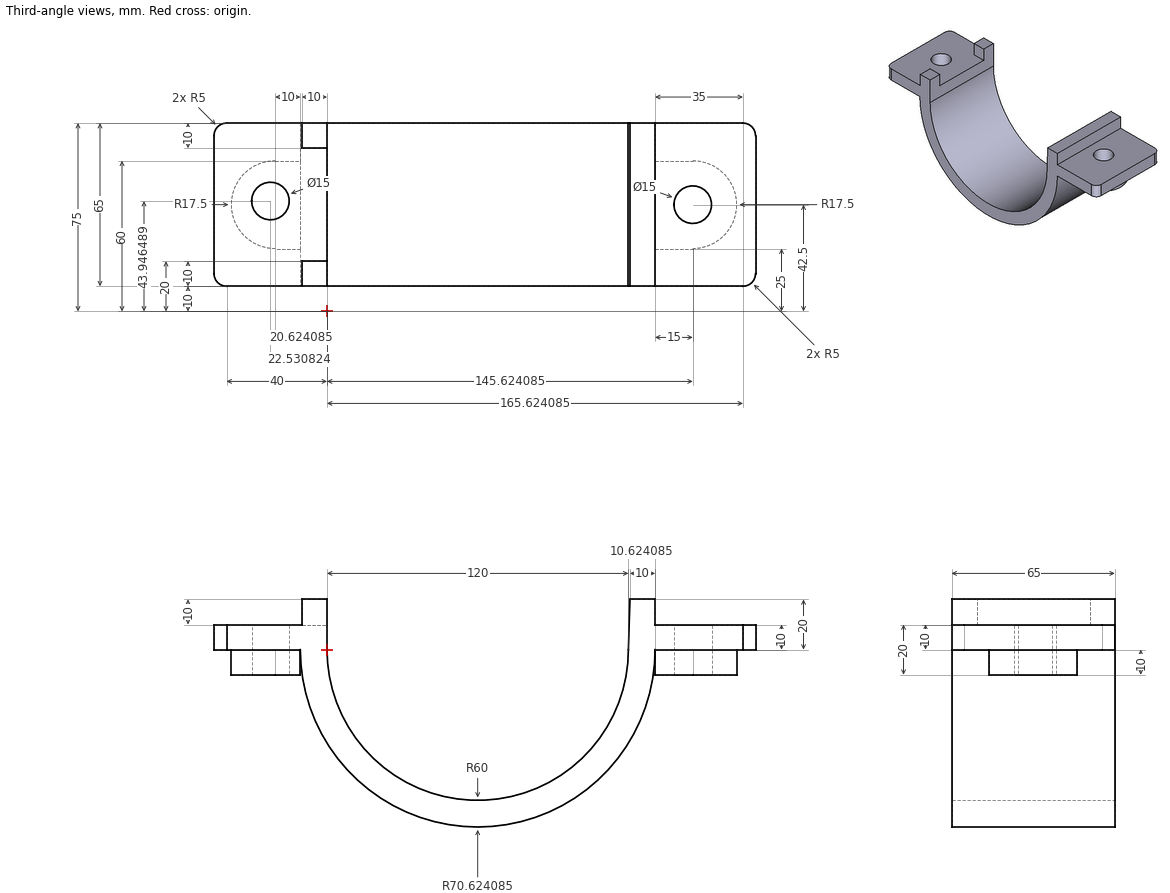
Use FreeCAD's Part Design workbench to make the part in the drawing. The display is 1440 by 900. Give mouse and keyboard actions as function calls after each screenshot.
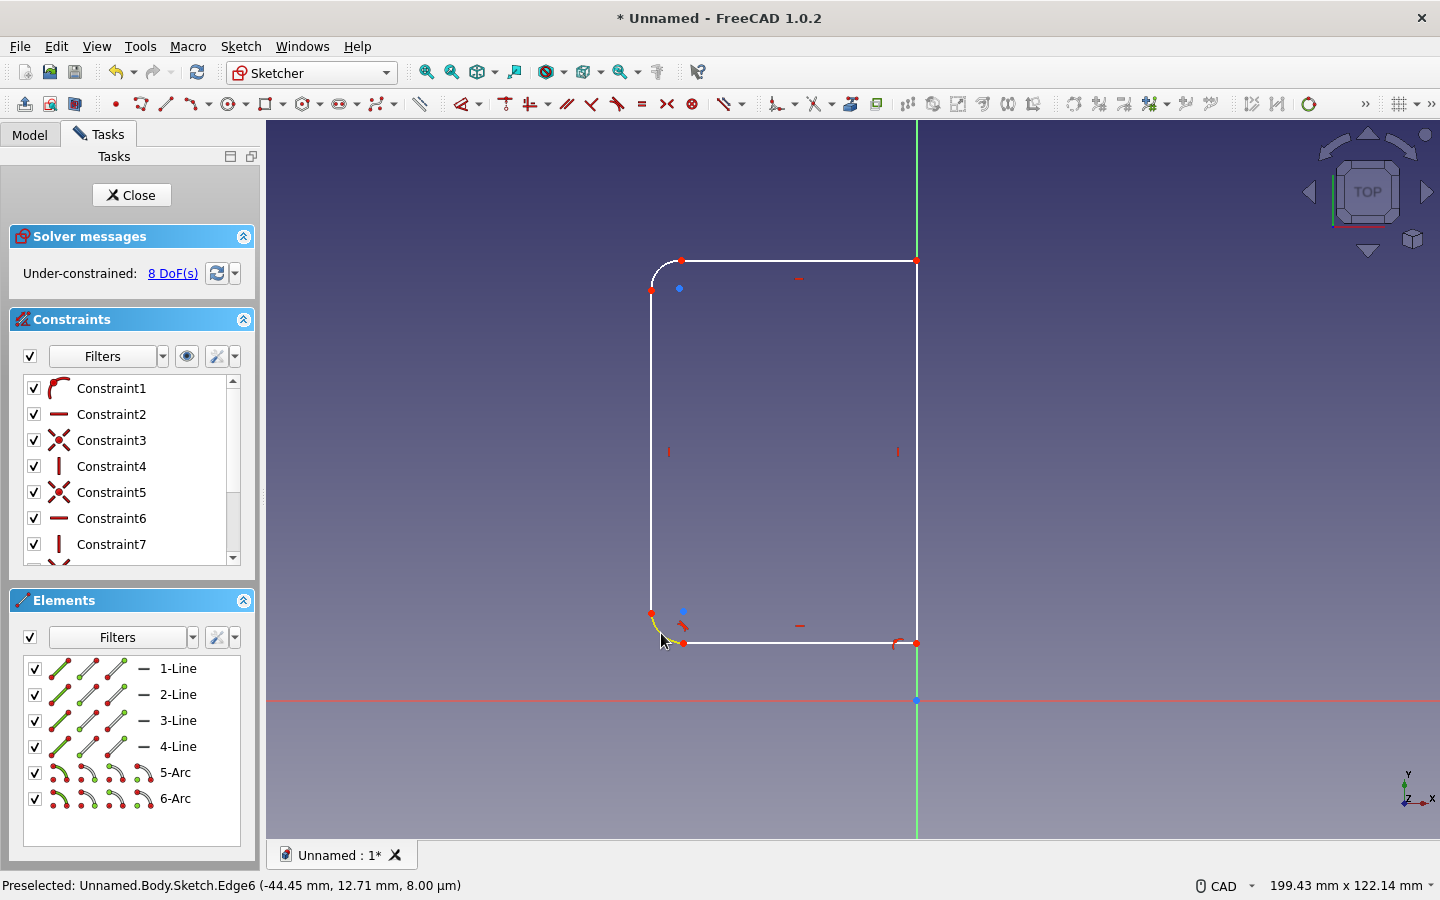
click(846, 261)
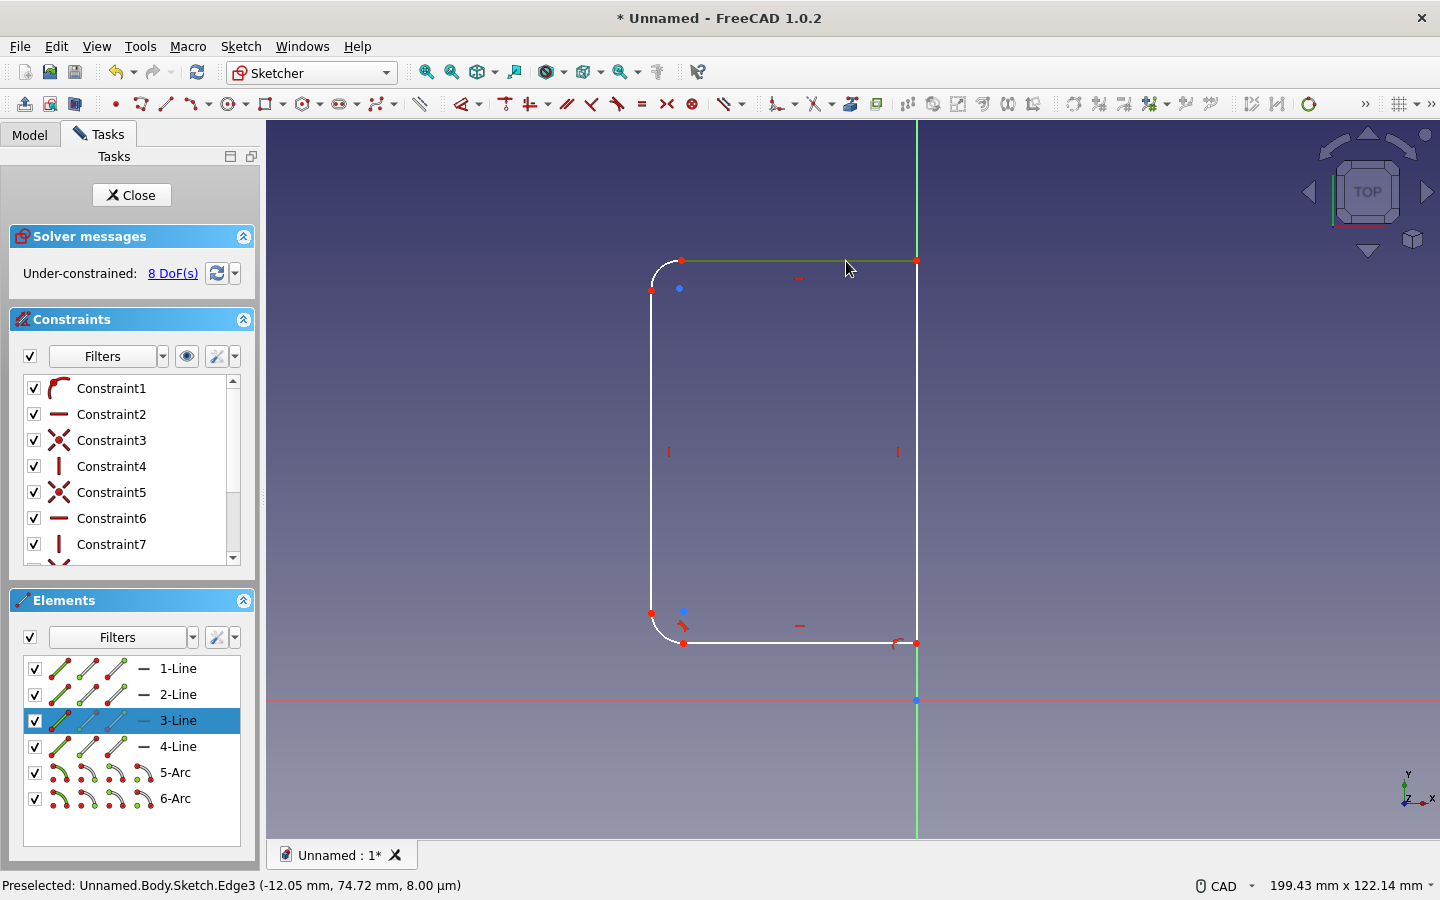
click(667, 263)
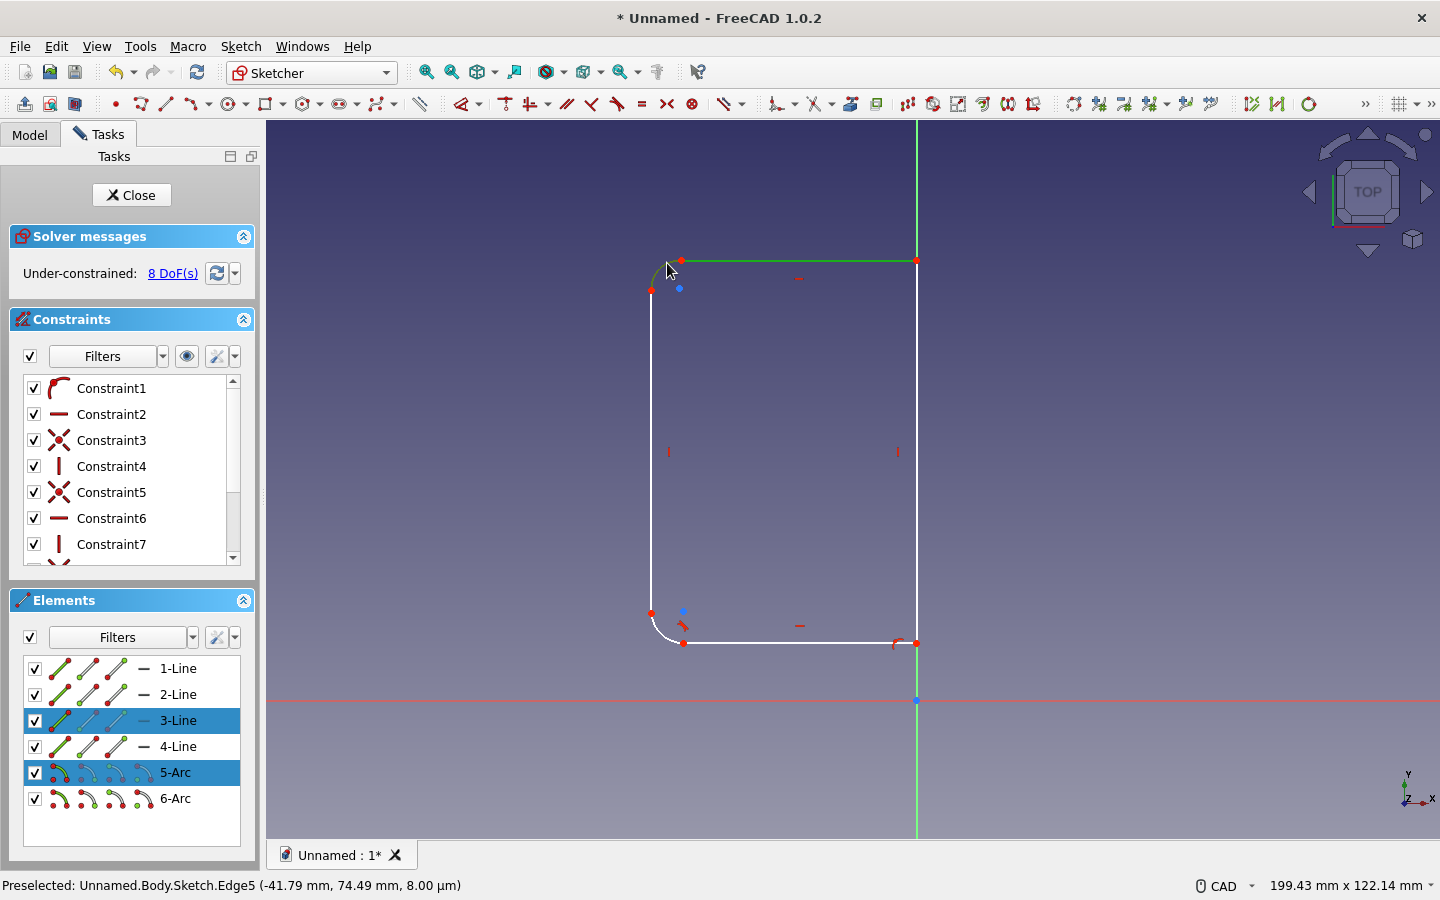
key(t)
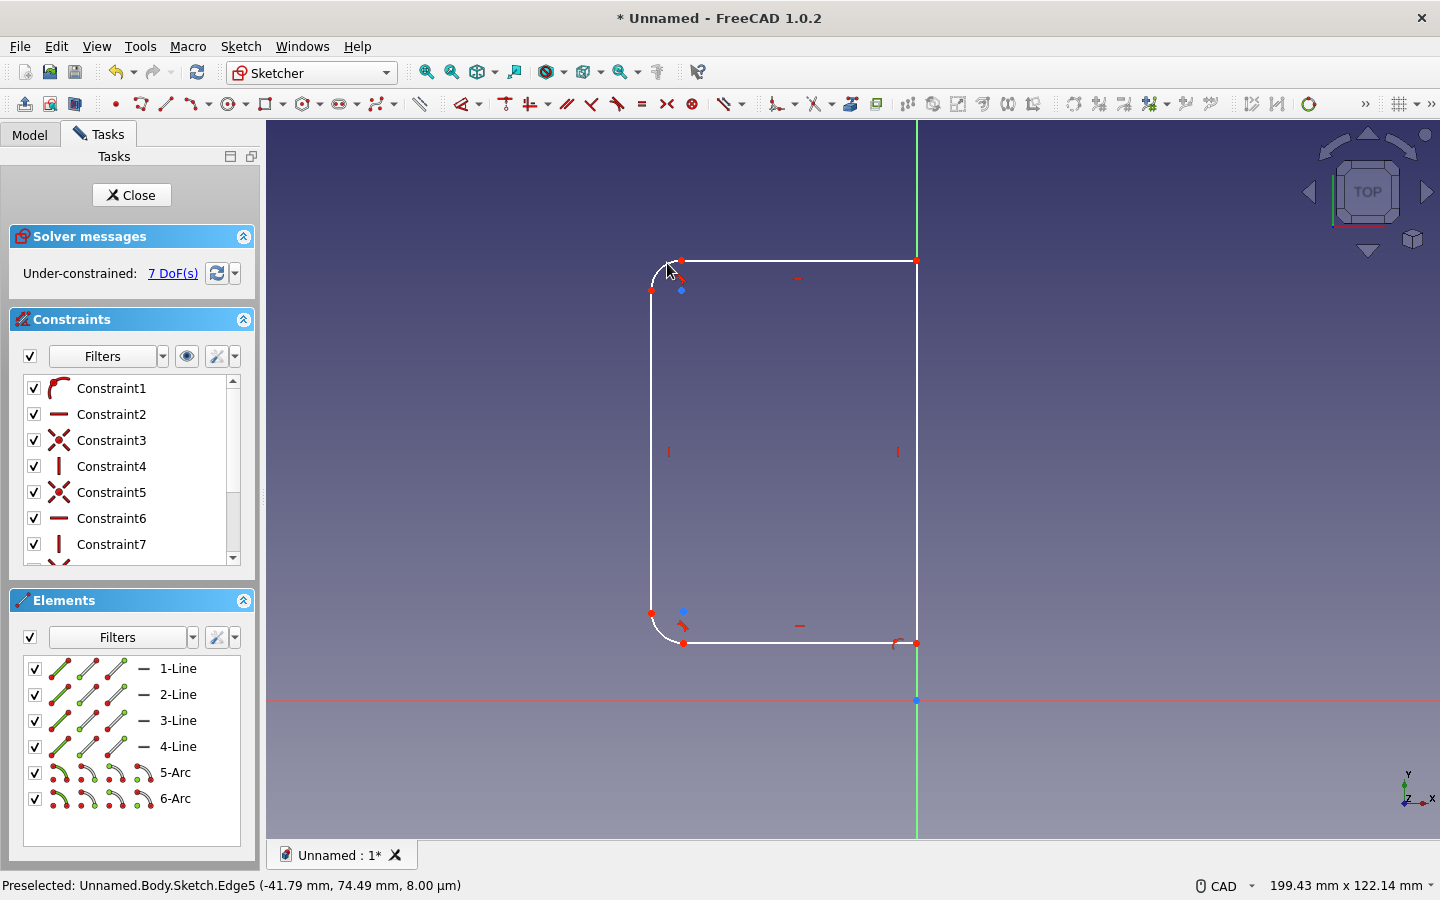
click(651, 387)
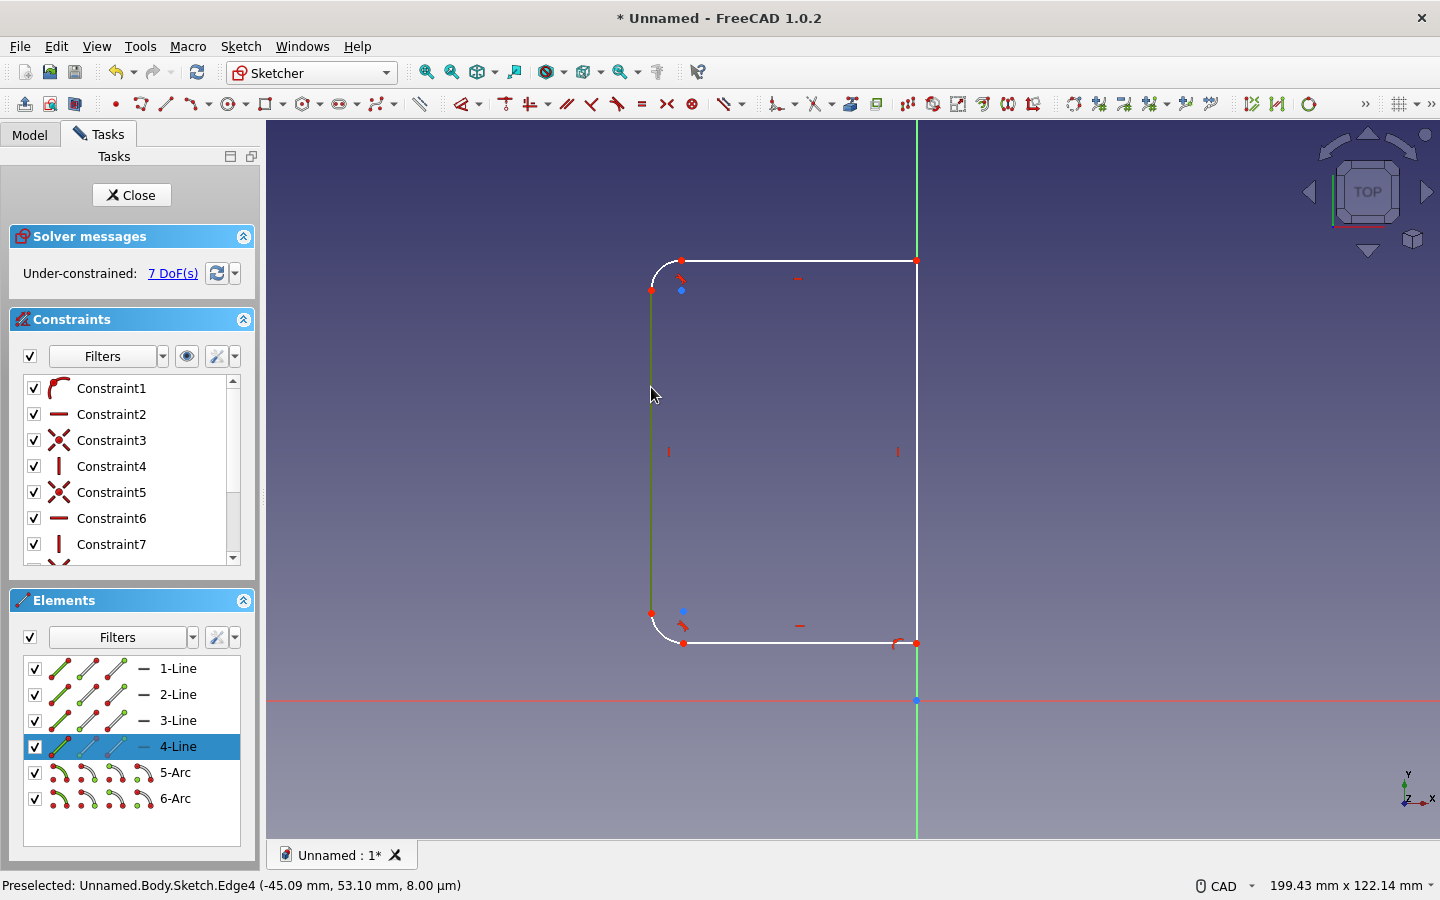
click(668, 264)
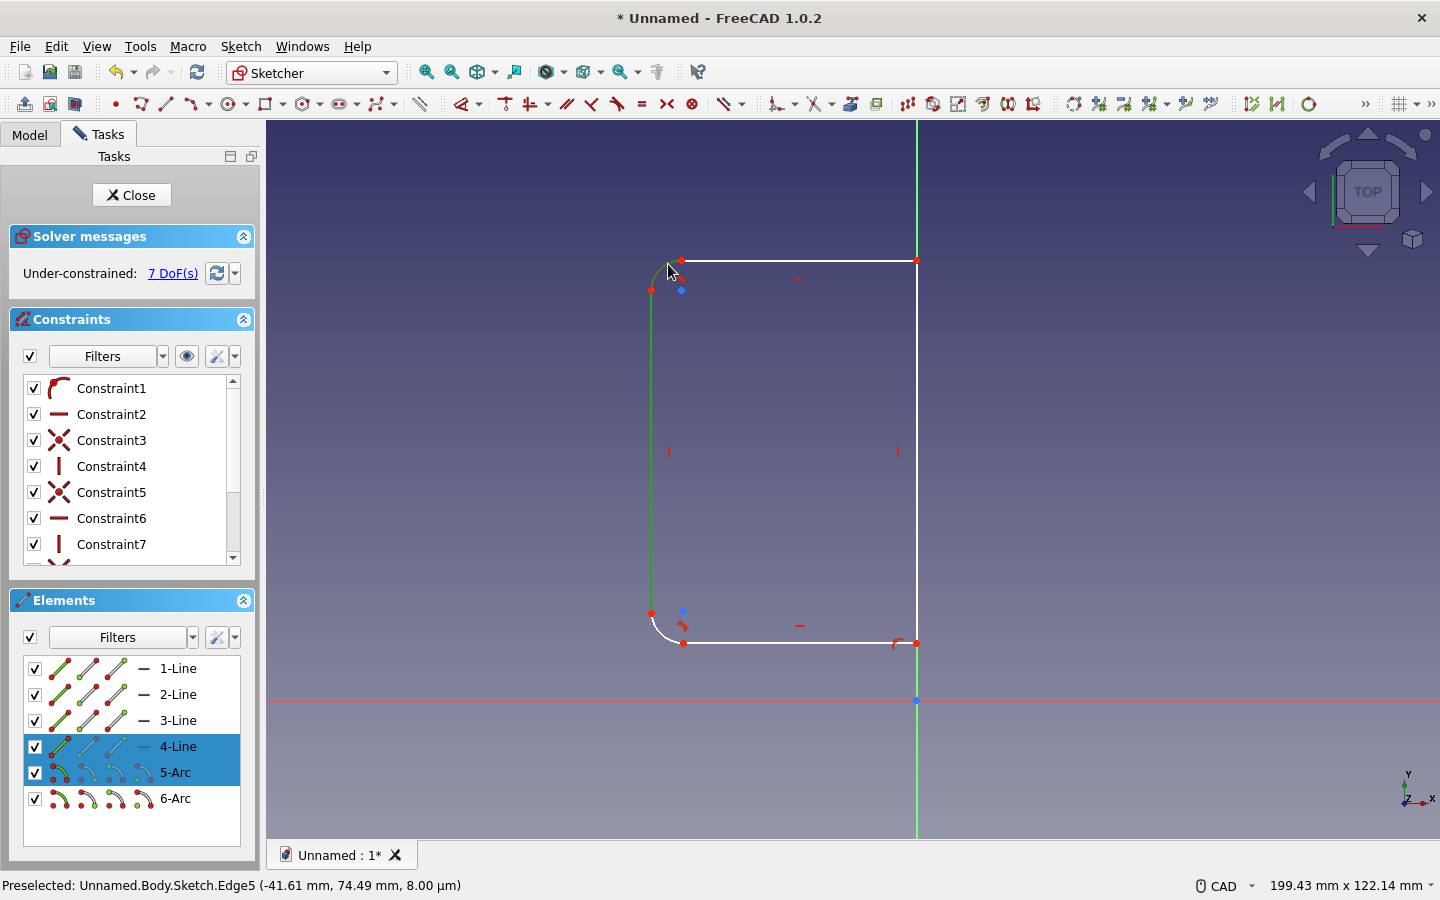
key(t)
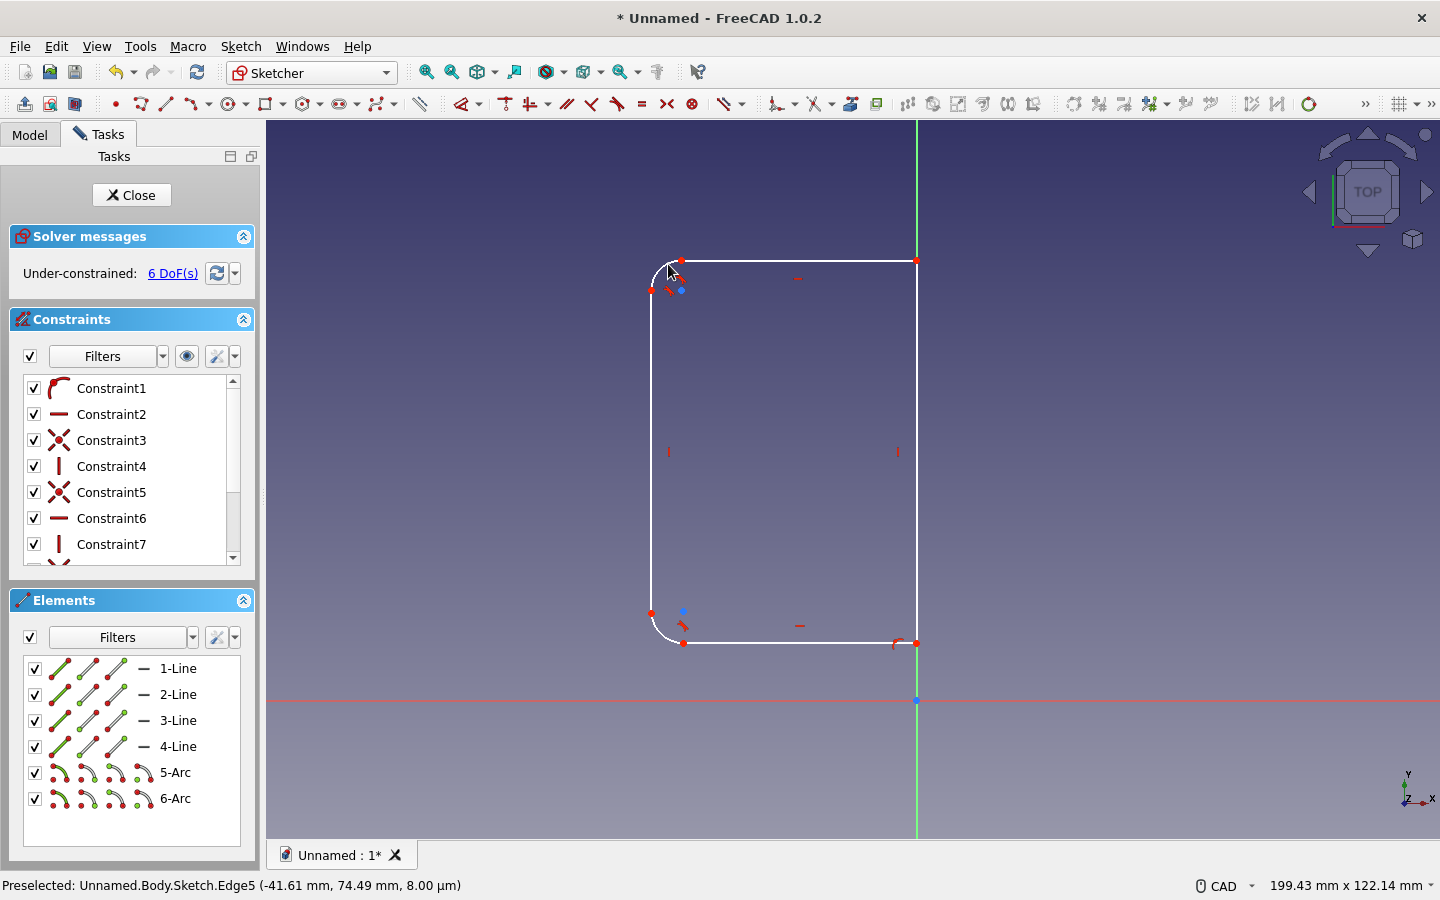
click(651, 387)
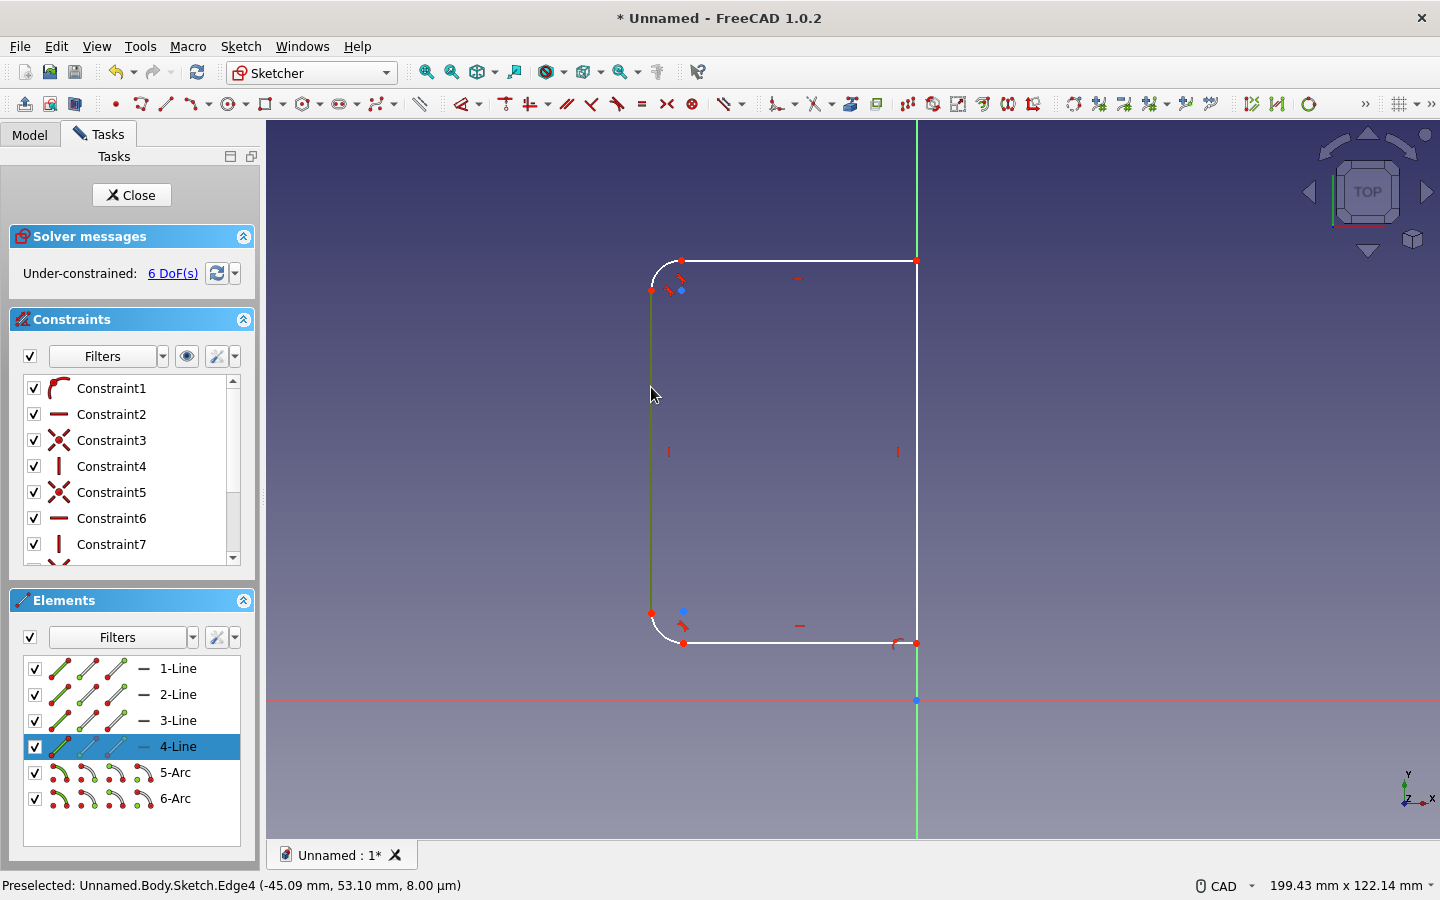
click(656, 627)